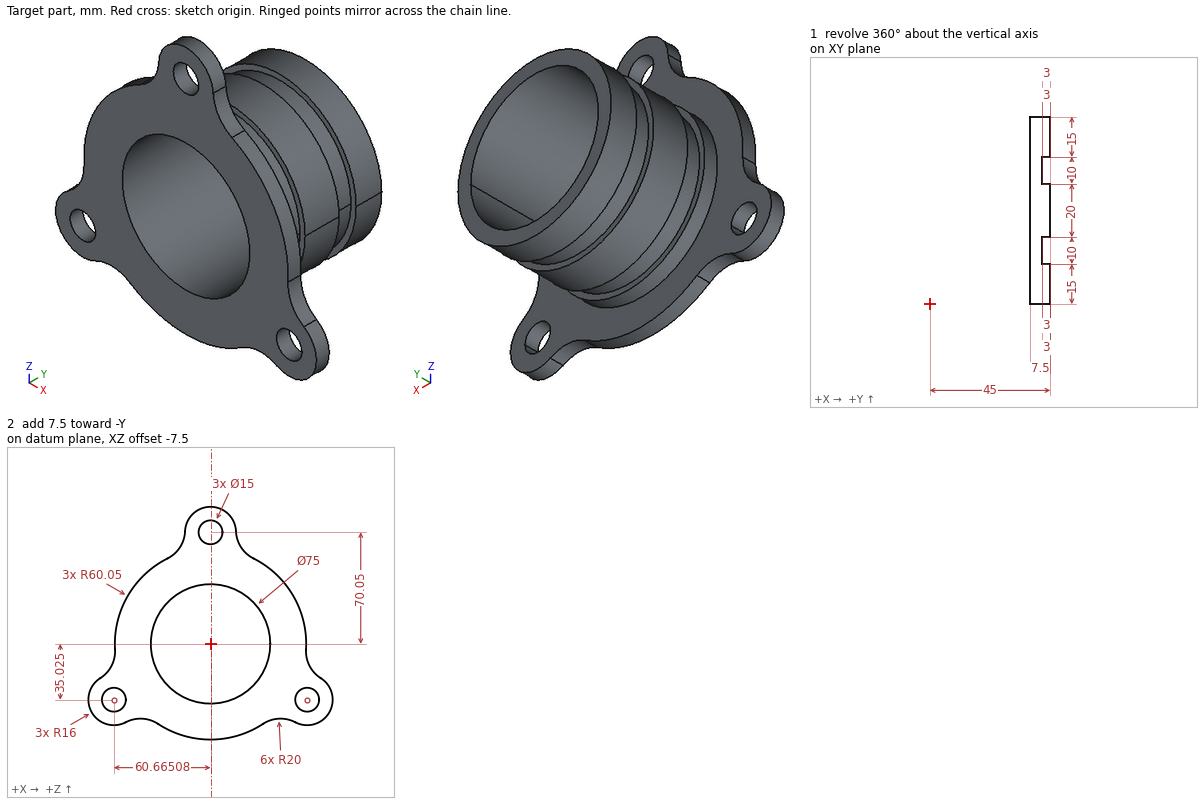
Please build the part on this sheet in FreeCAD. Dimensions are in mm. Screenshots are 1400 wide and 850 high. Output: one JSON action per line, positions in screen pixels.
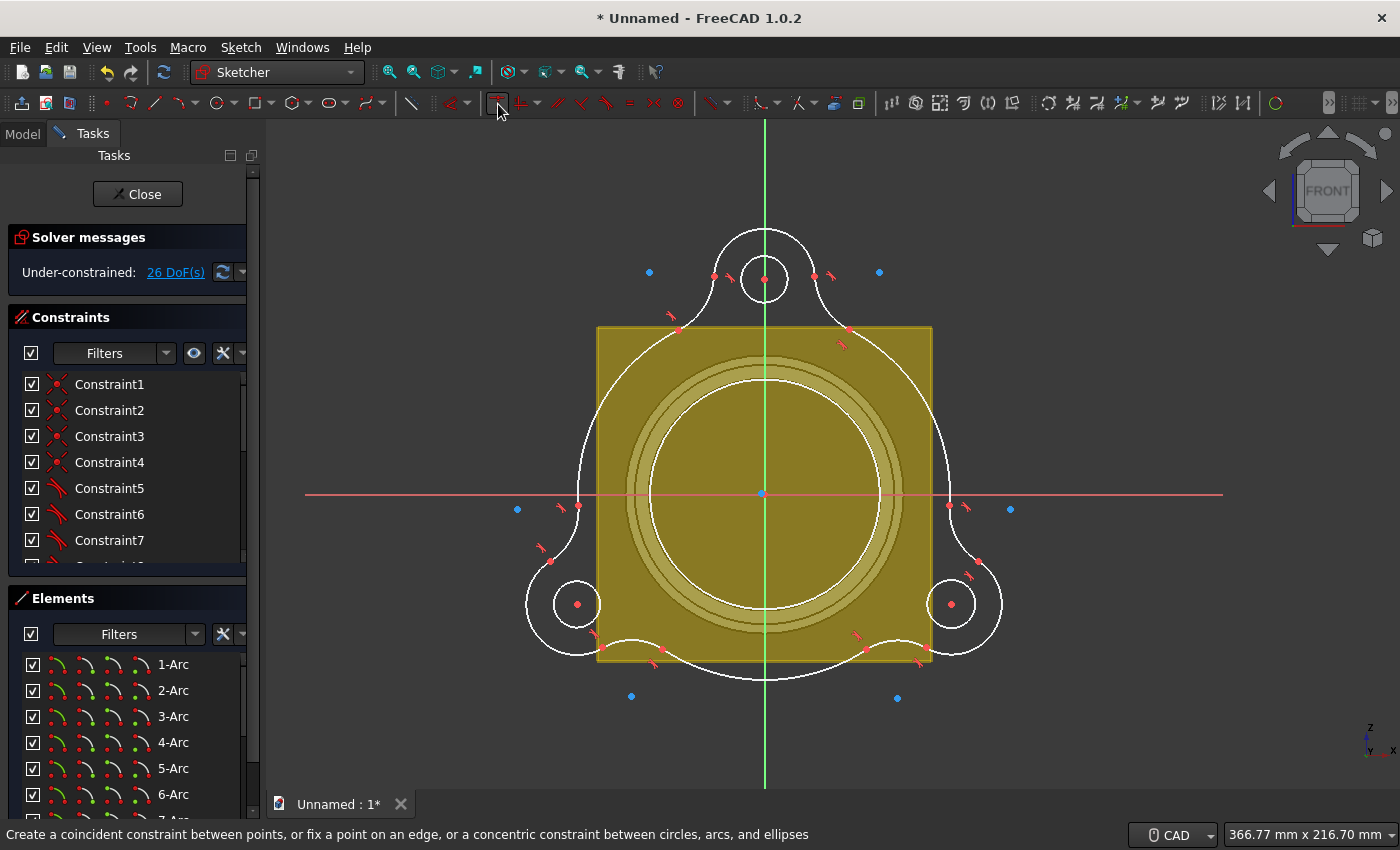
{"action": "left_click", "coordinate": [846, 413]}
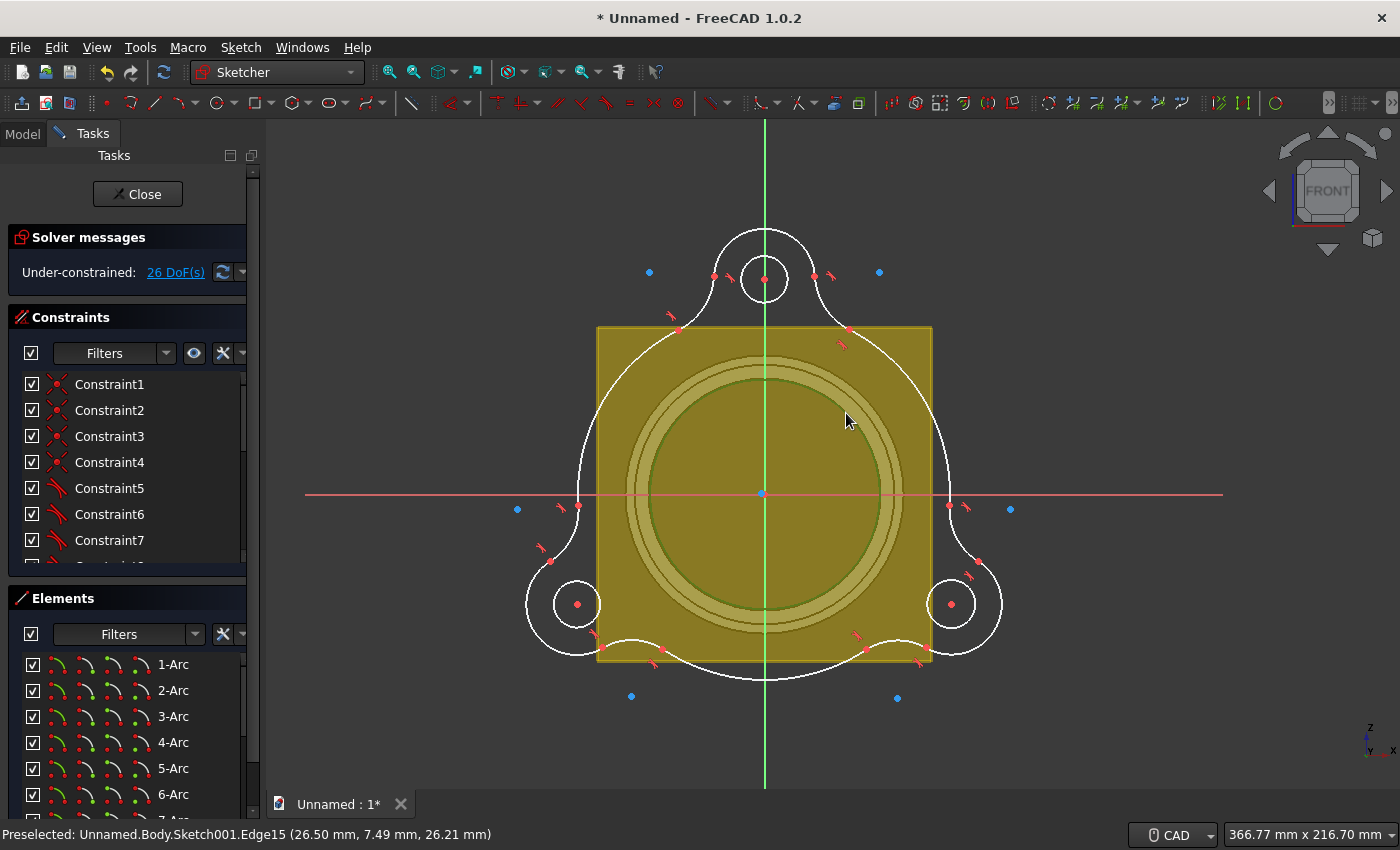
{"action": "left_click", "coordinate": [627, 368]}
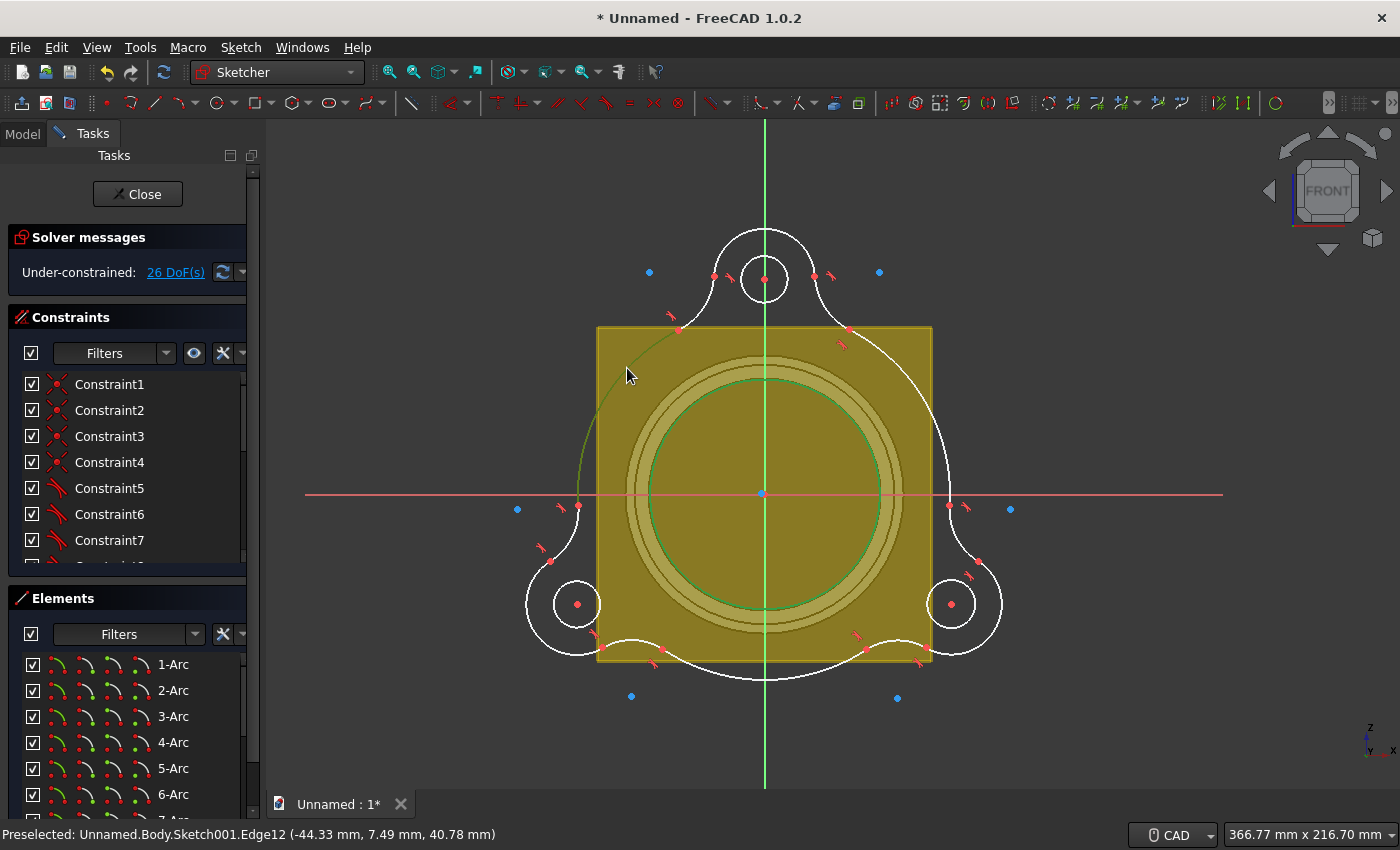
{"action": "left_click", "coordinate": [498, 104]}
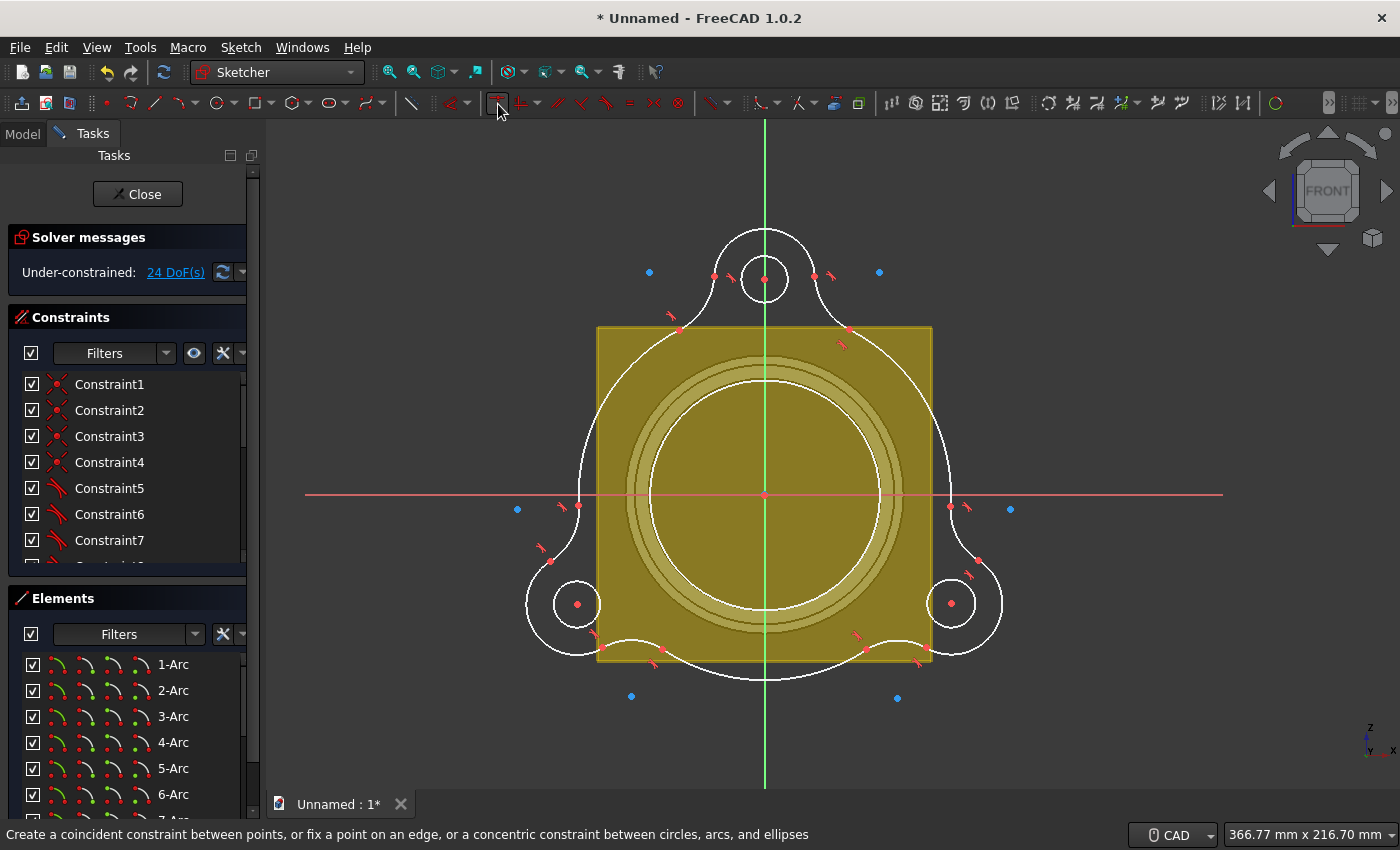
{"action": "scroll", "coordinate": [765, 495], "scroll_direction": "up", "scroll_amount": 3}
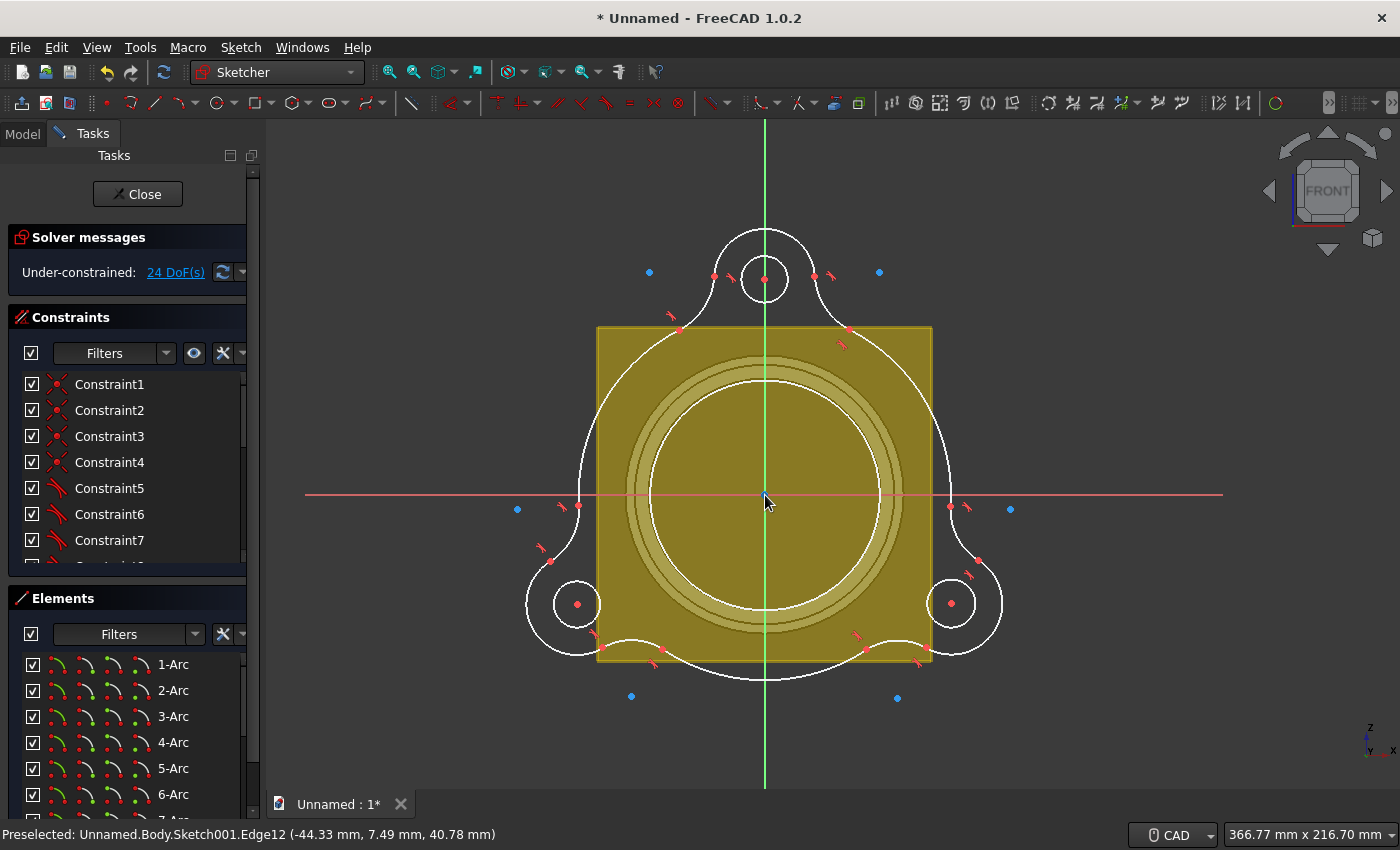
{"action": "left_click_drag", "start_coordinate": [754, 484], "coordinate": [775, 505]}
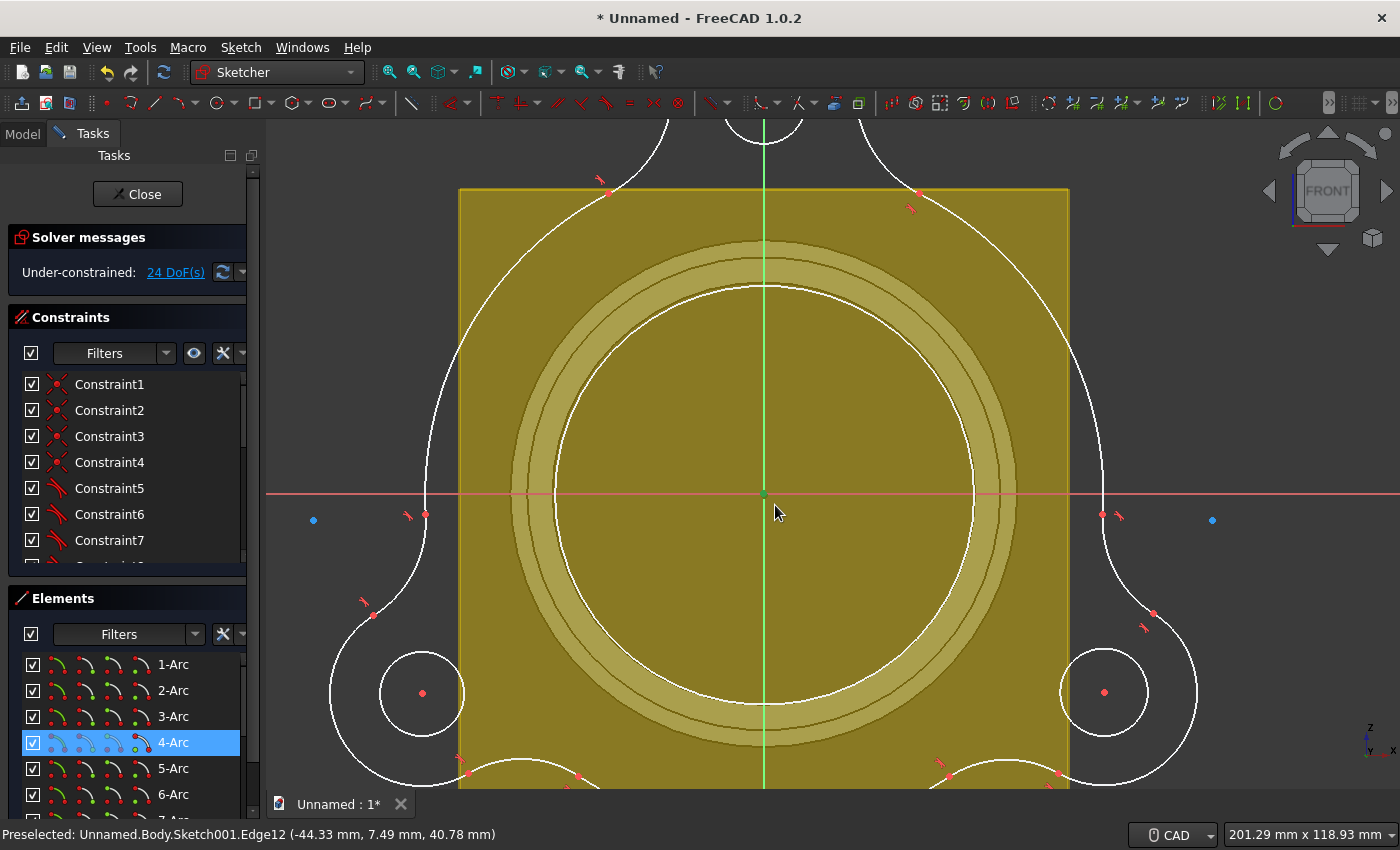
{"action": "left_click", "coordinate": [498, 104]}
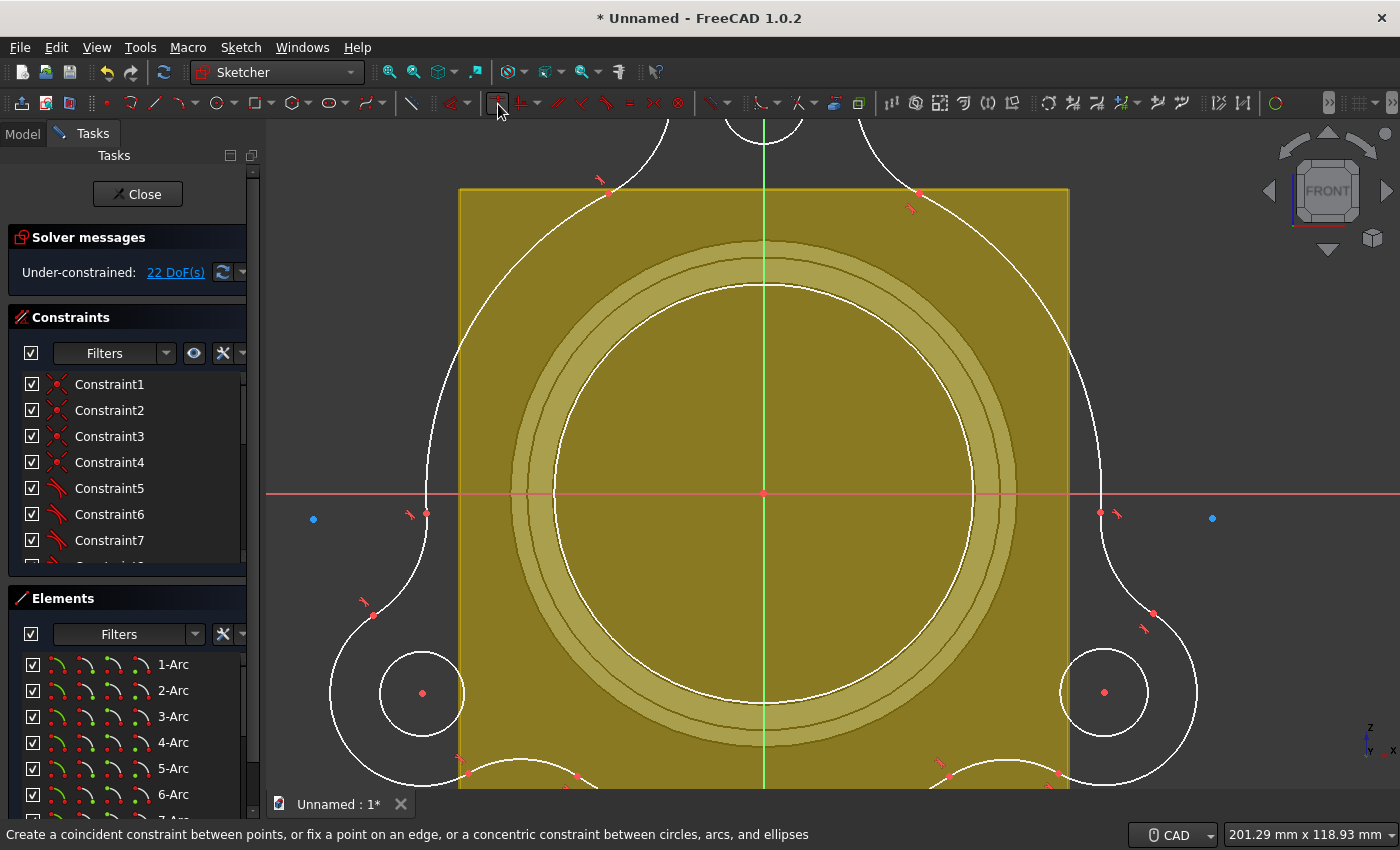
{"action": "left_click", "coordinate": [401, 592]}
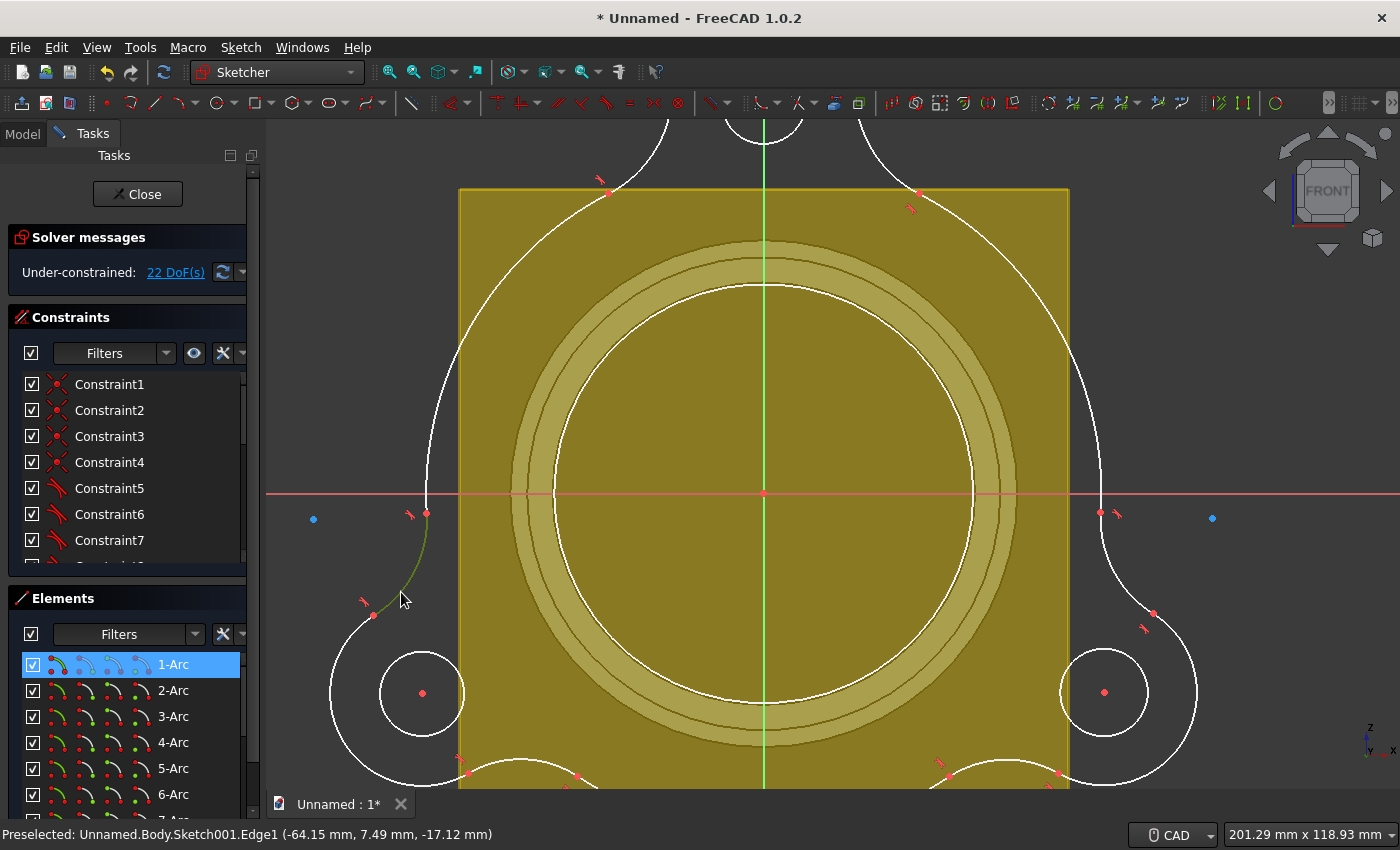
{"action": "left_click", "coordinate": [523, 759]}